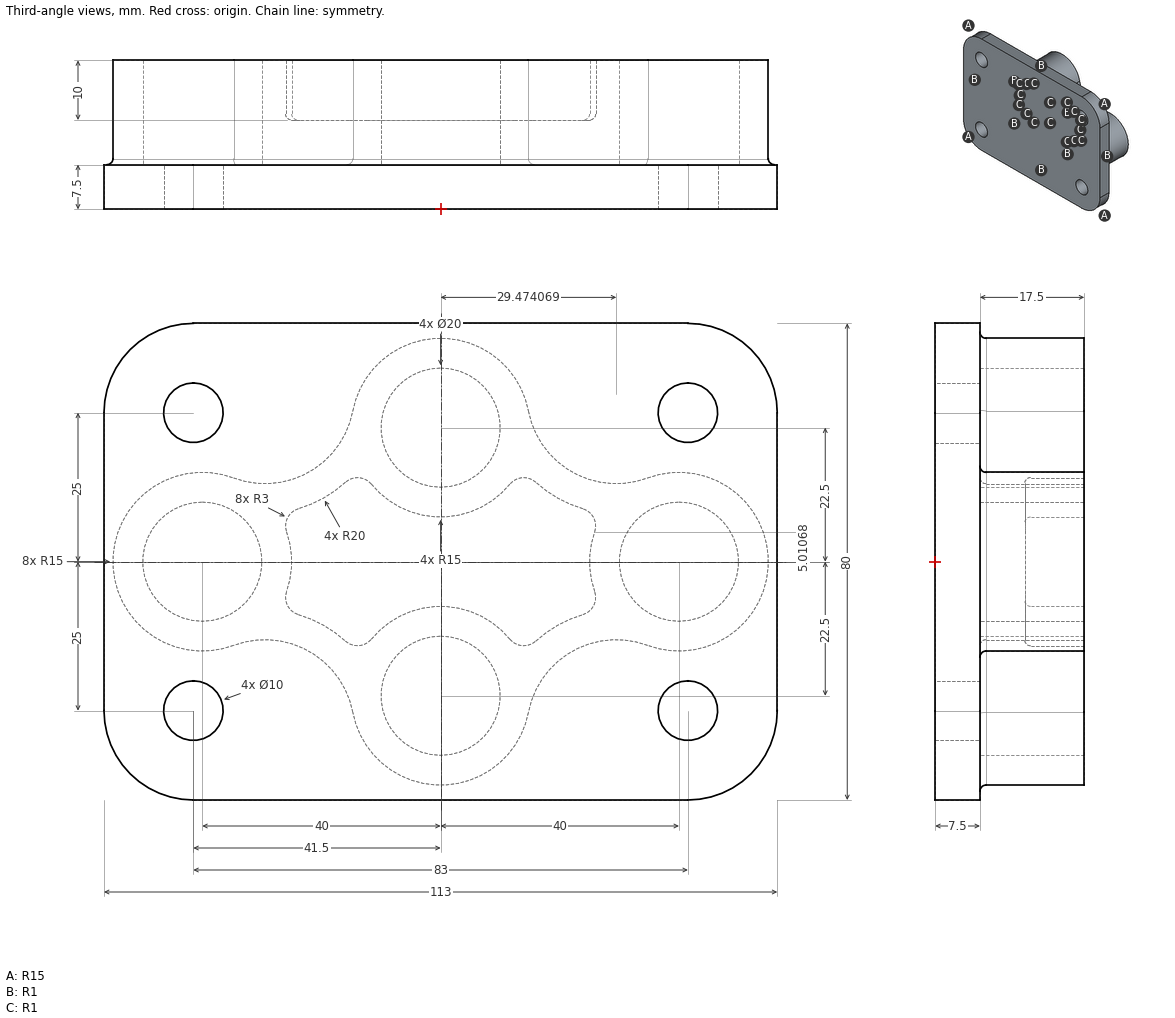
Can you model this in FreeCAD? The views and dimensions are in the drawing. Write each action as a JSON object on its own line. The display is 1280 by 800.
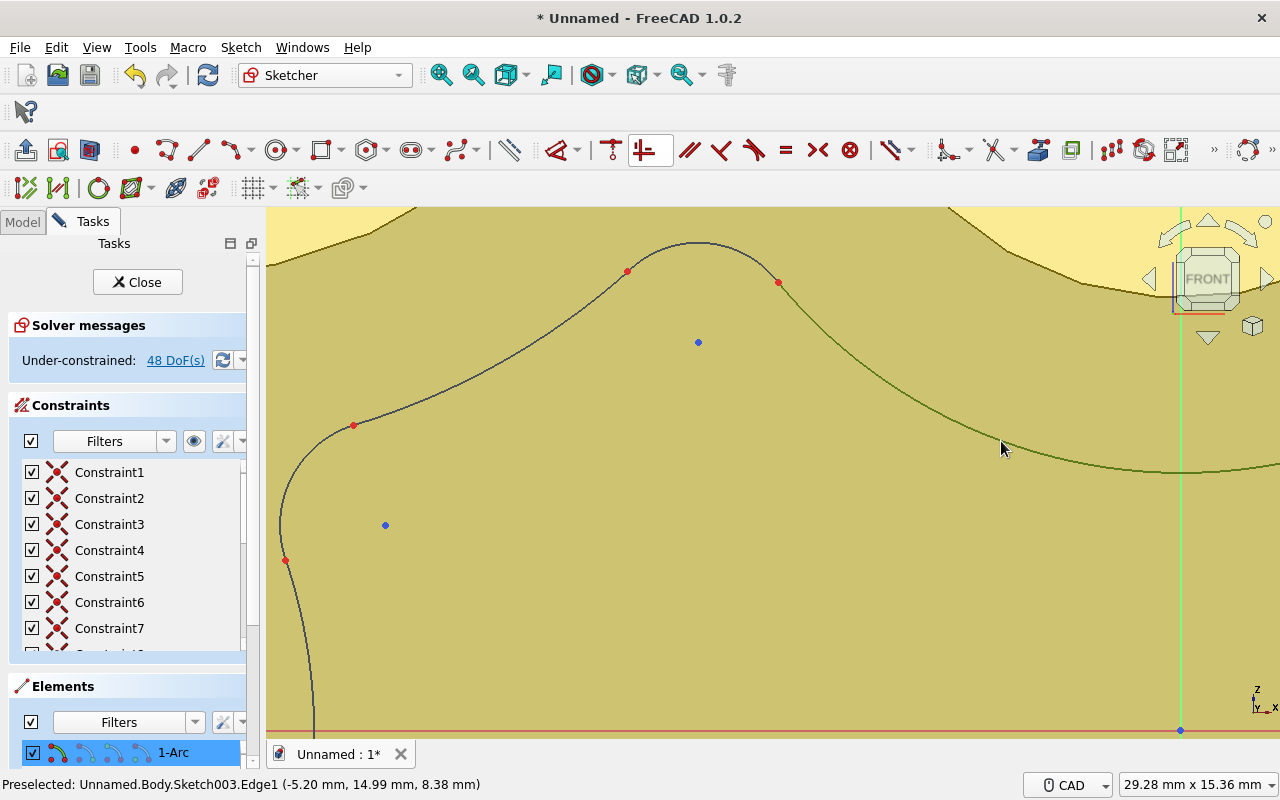
{"action": "scroll", "coordinate": [499, 362], "scroll_direction": "down", "scroll_amount": 6}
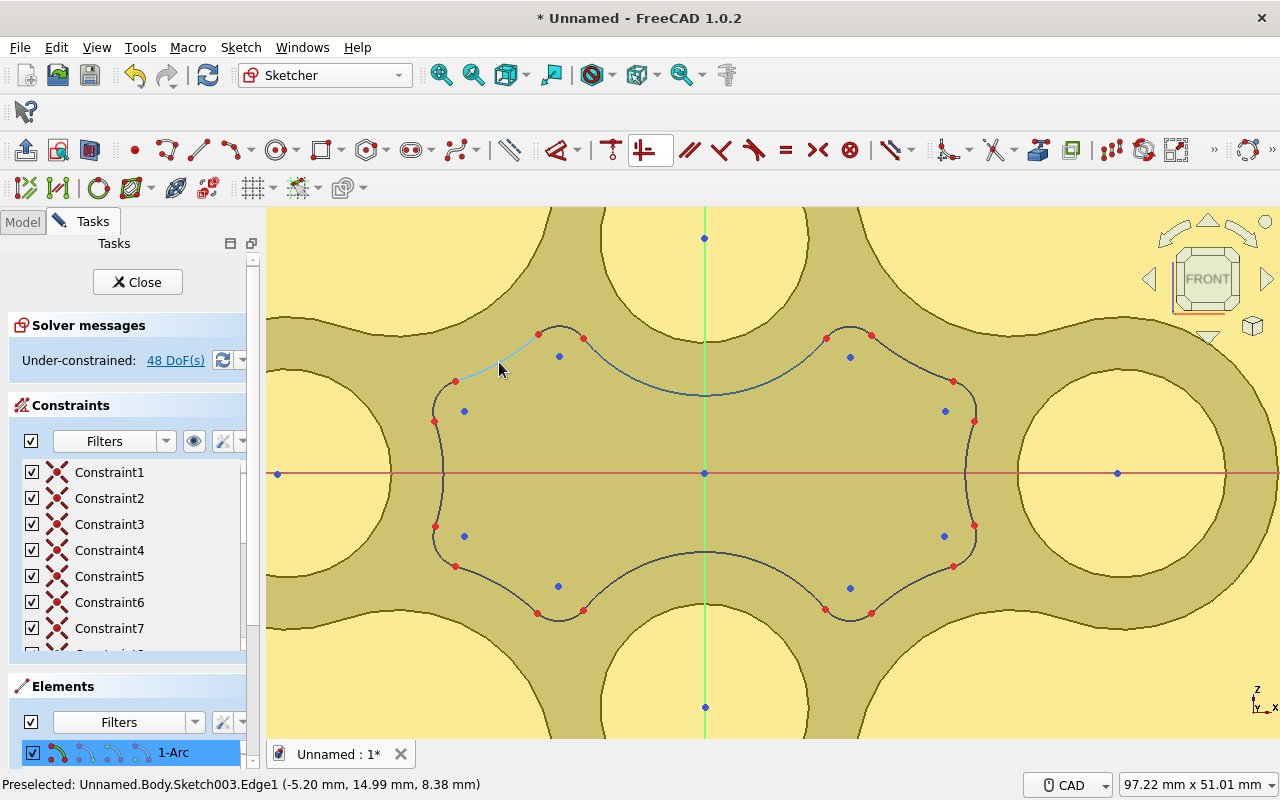
{"action": "left_click", "coordinate": [858, 328]}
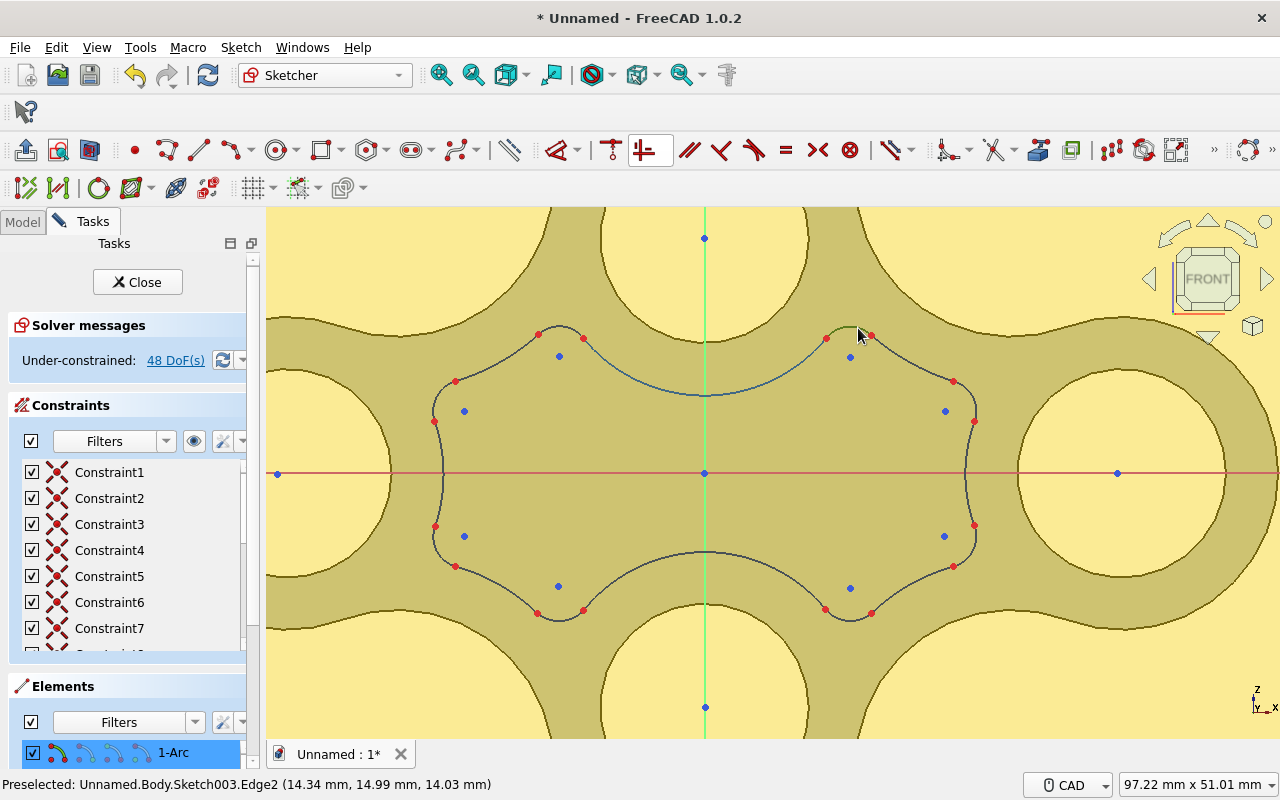
{"action": "left_click", "coordinate": [754, 150]}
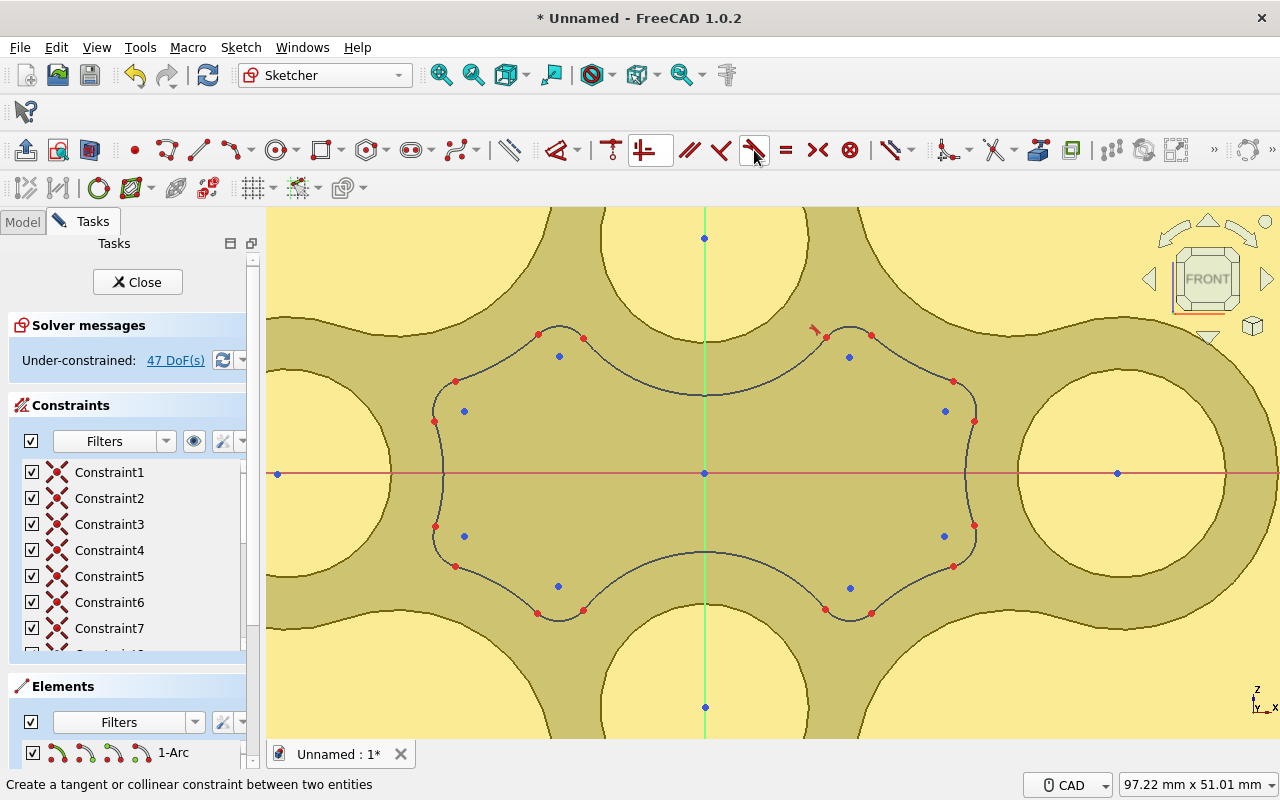
{"action": "left_click", "coordinate": [650, 386]}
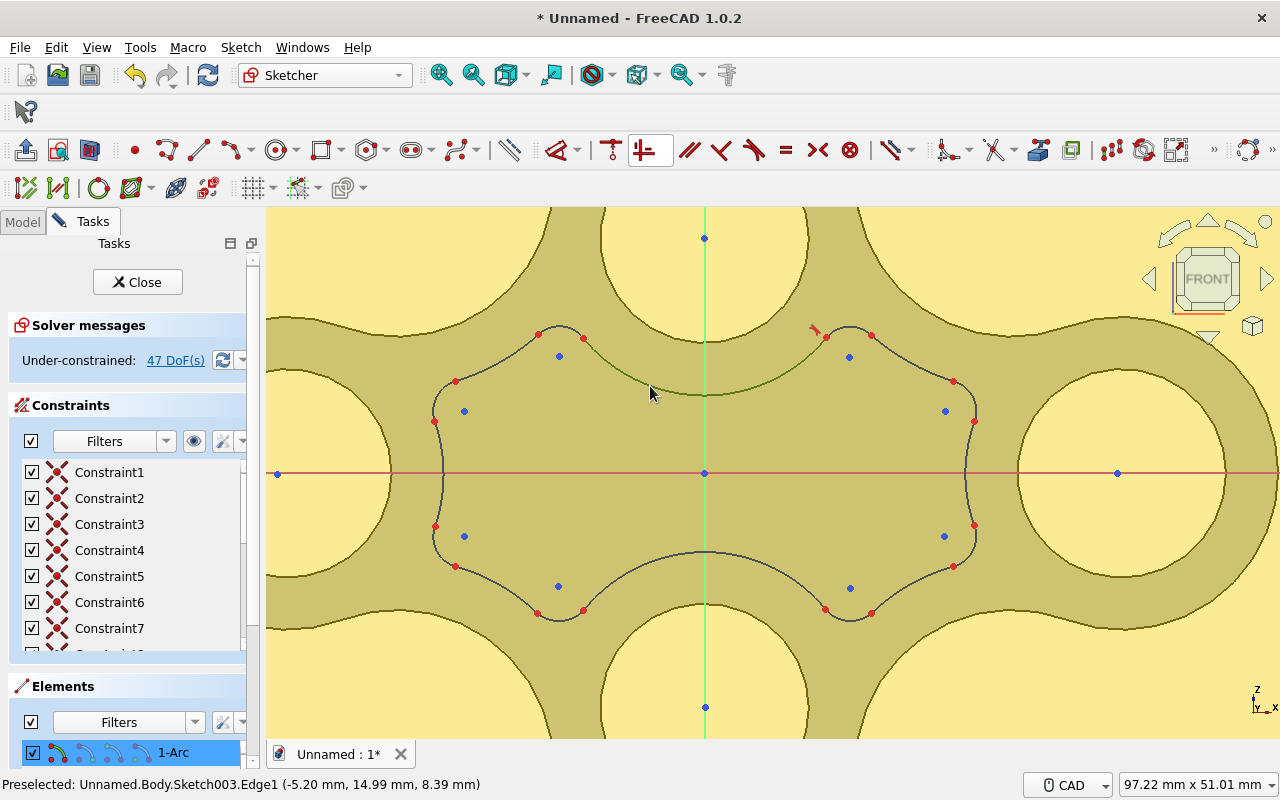
{"action": "left_click", "coordinate": [571, 329]}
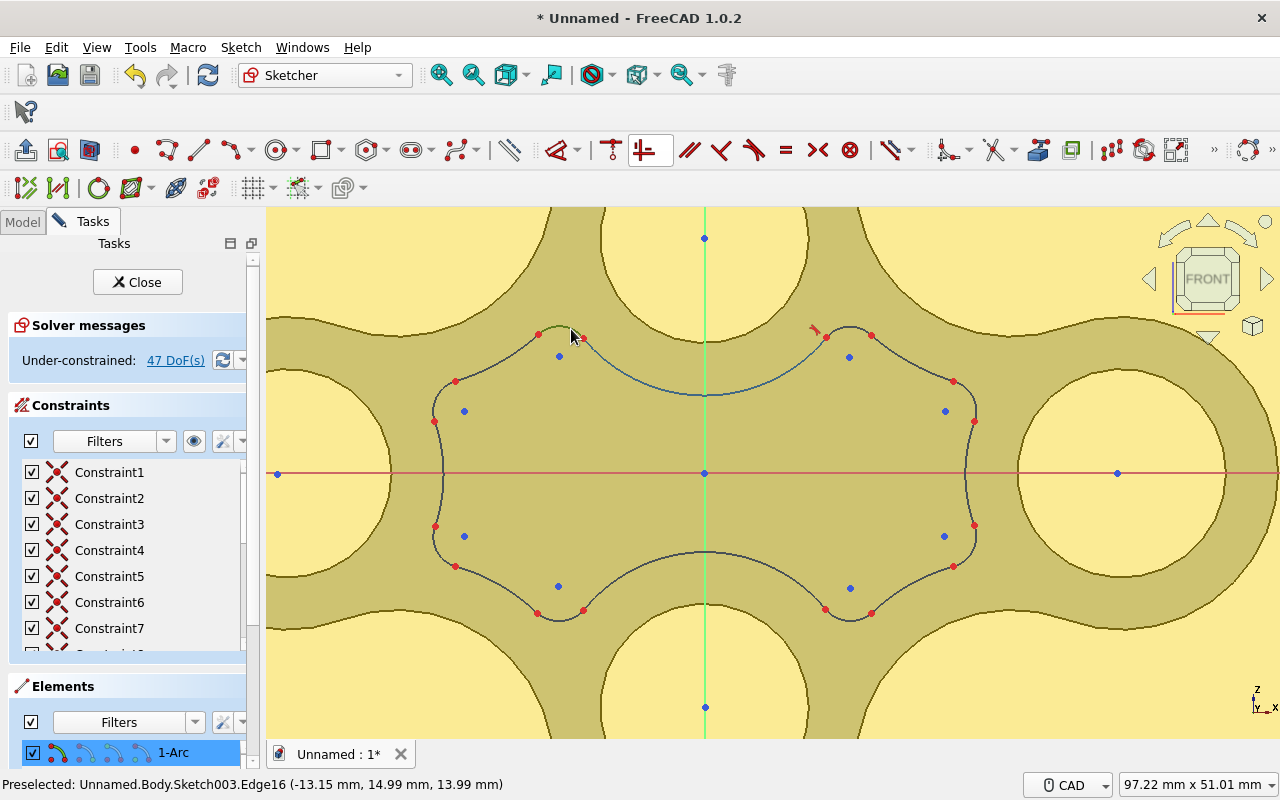
{"action": "key", "text": "t"}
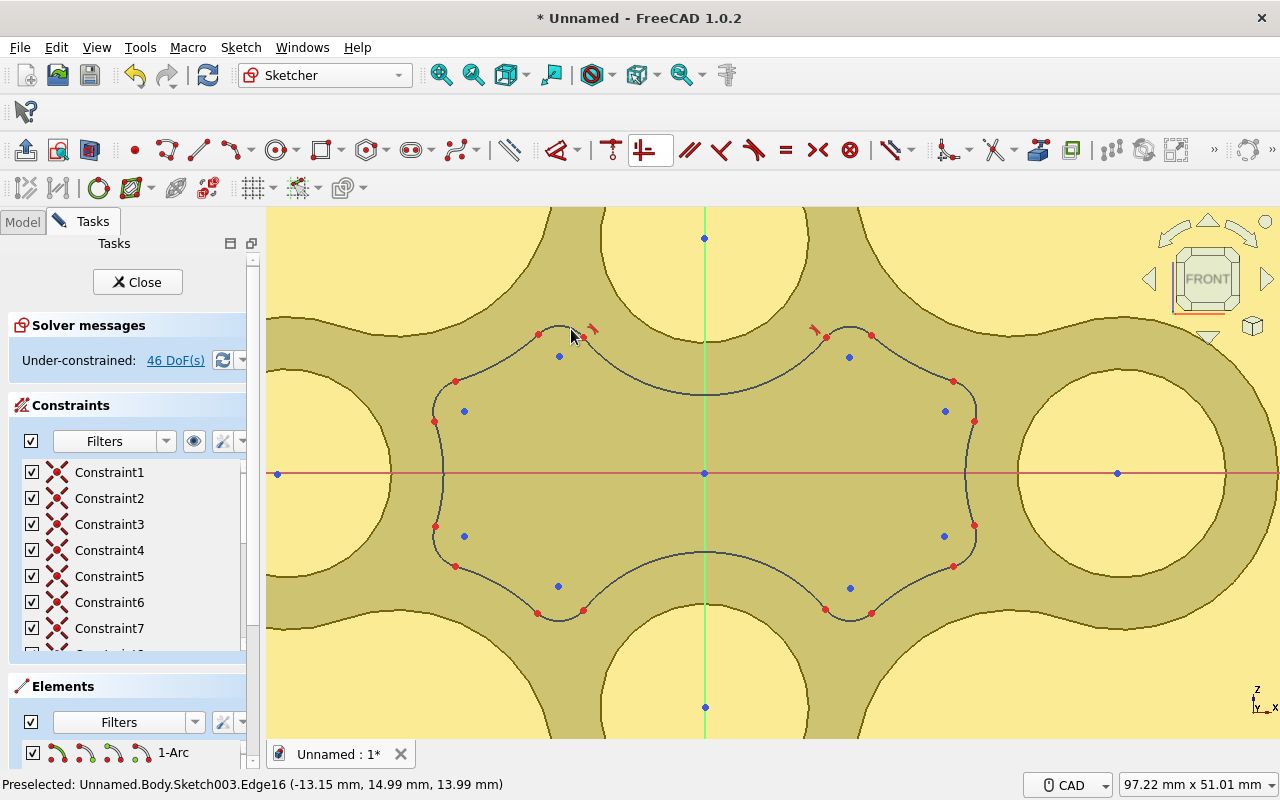
{"action": "left_click", "coordinate": [858, 328]}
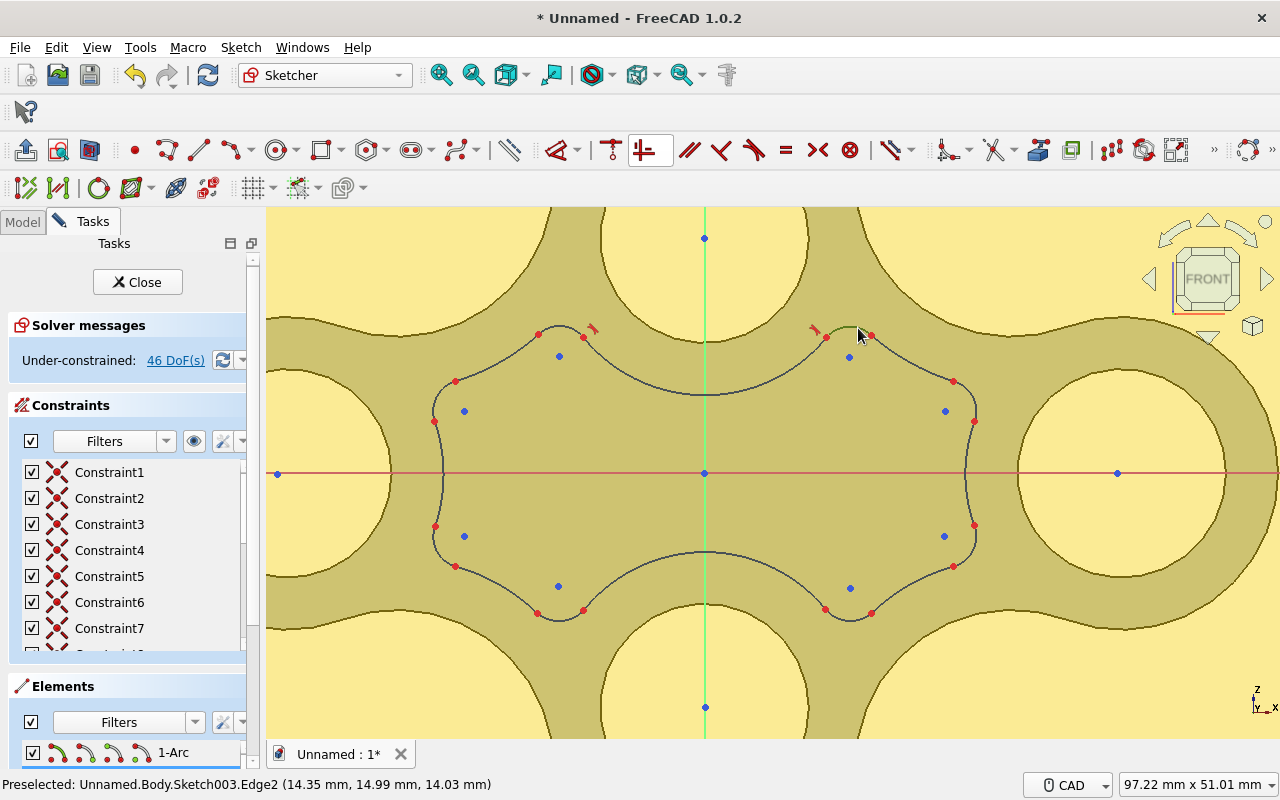
{"action": "left_click", "coordinate": [894, 352]}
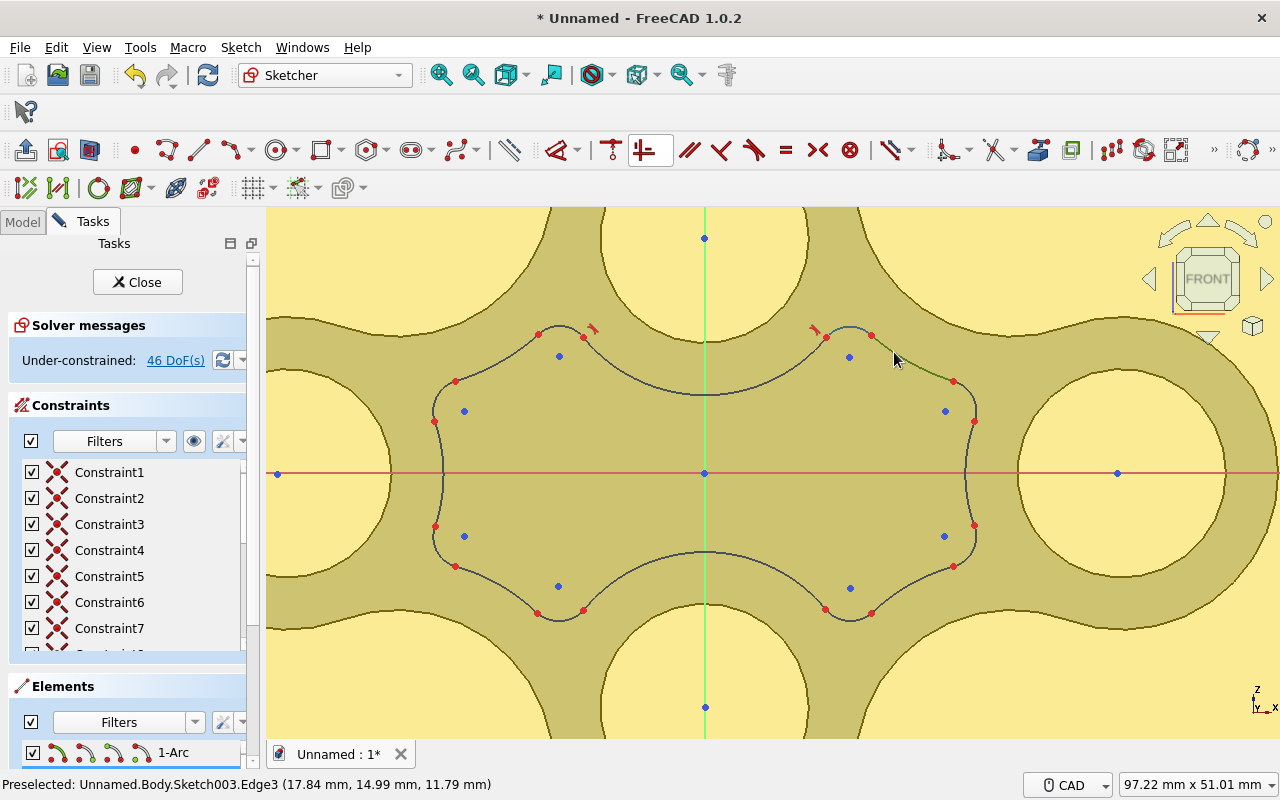
{"action": "key", "text": "t"}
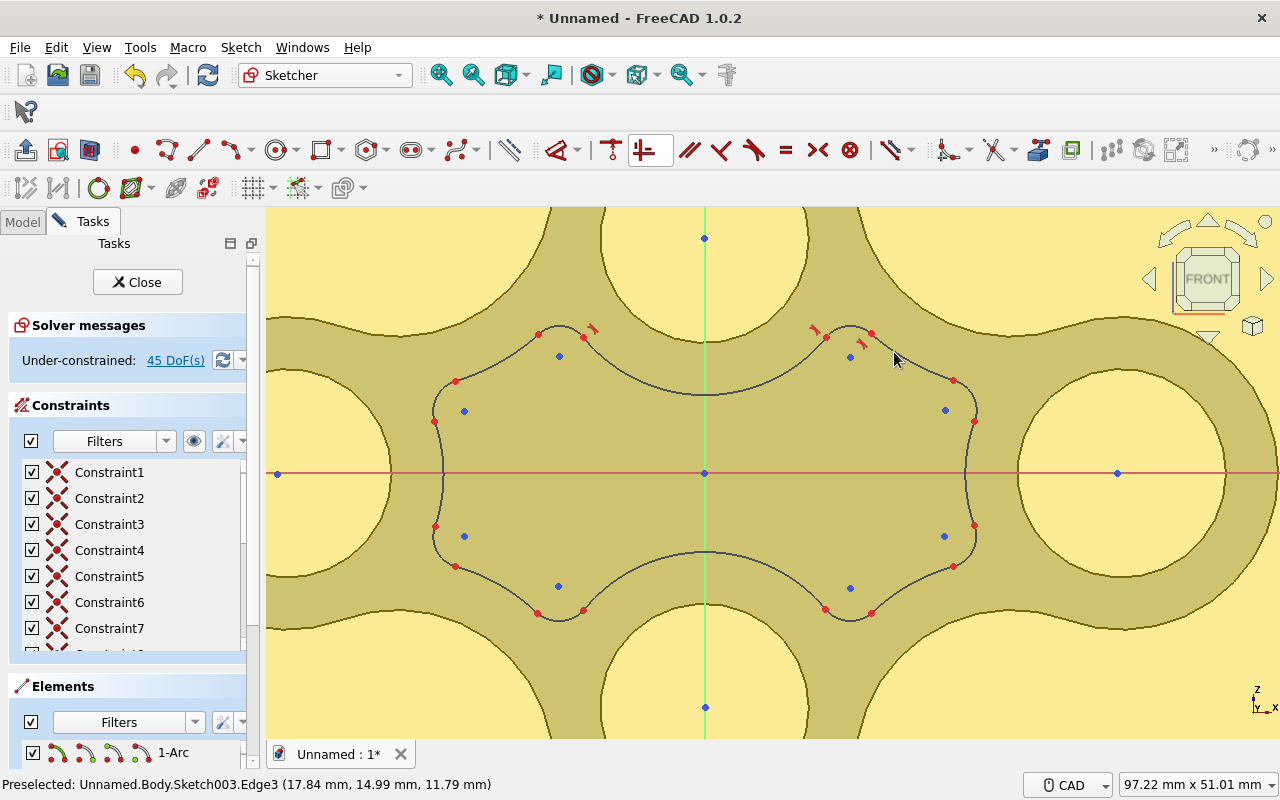
{"action": "left_click", "coordinate": [894, 351]}